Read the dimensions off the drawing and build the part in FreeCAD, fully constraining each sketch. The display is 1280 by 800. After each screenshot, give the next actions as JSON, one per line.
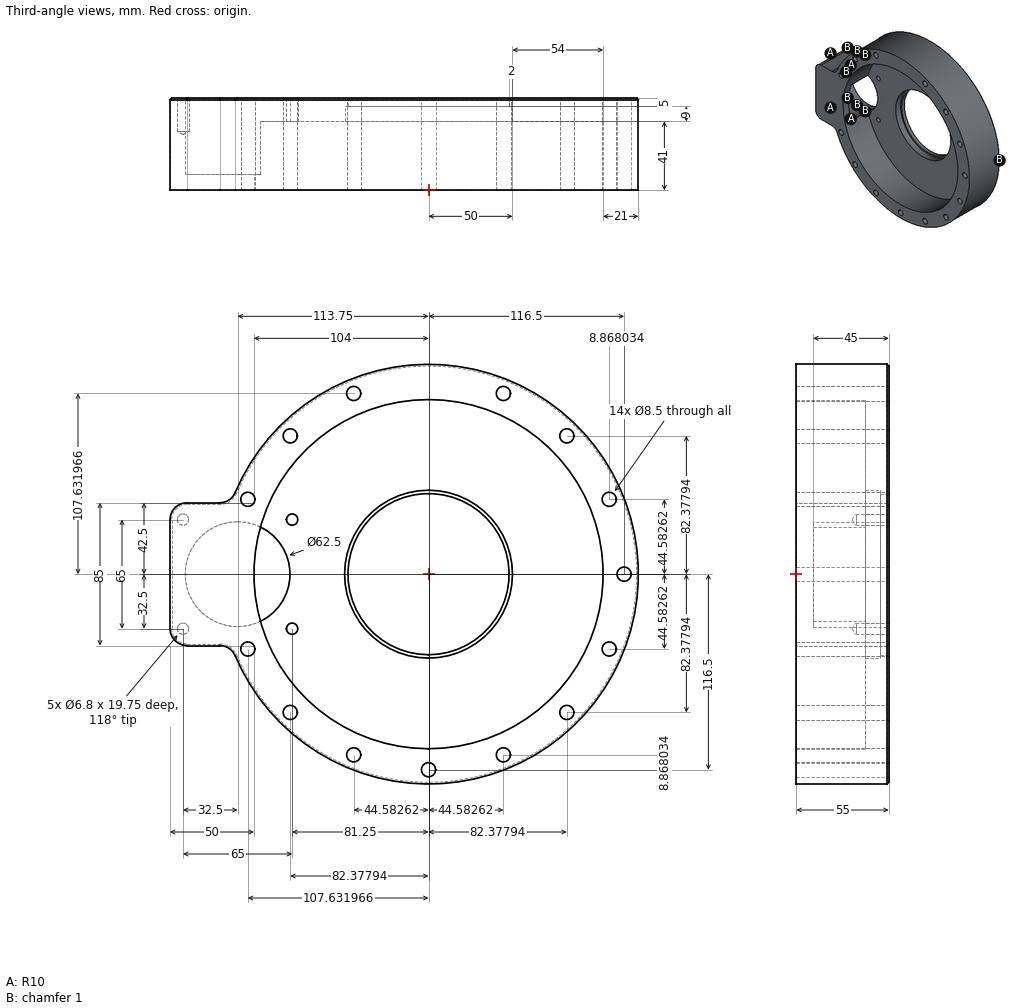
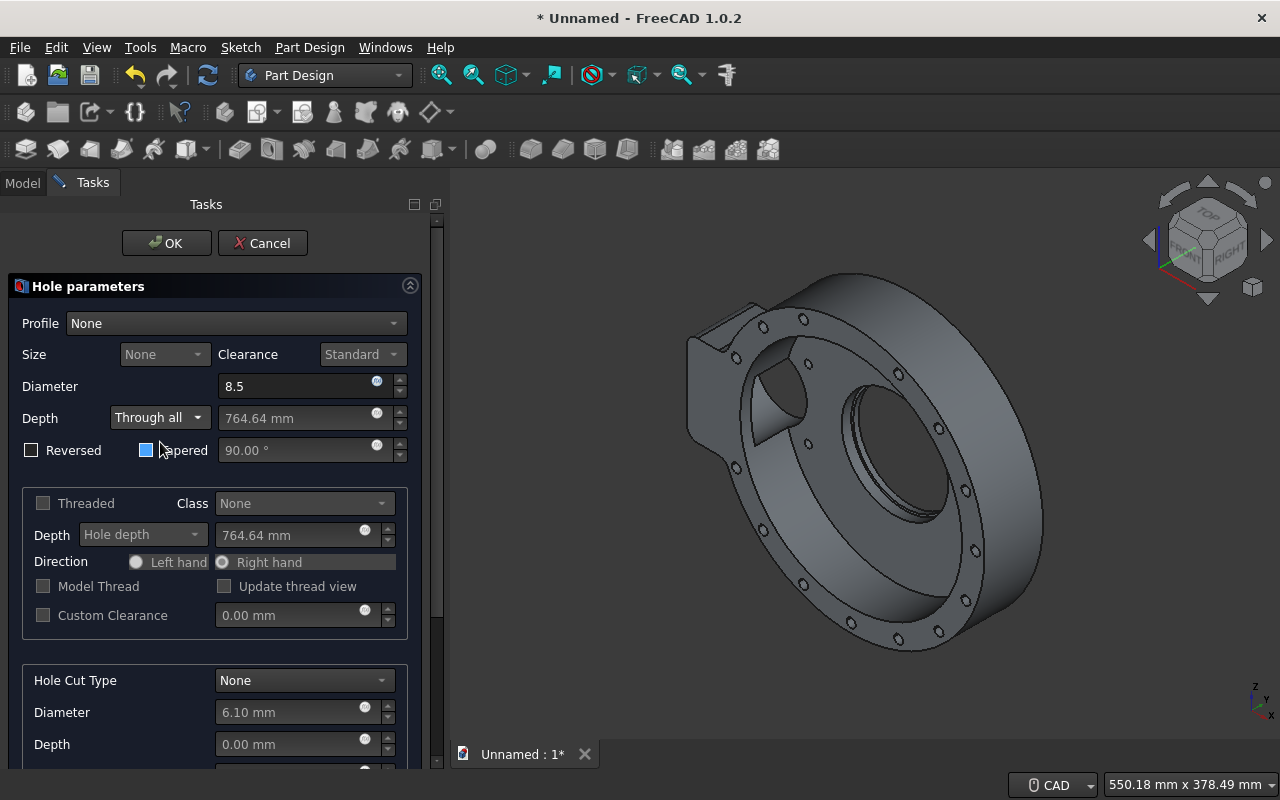
{"action": "left_click", "coordinate": [167, 243]}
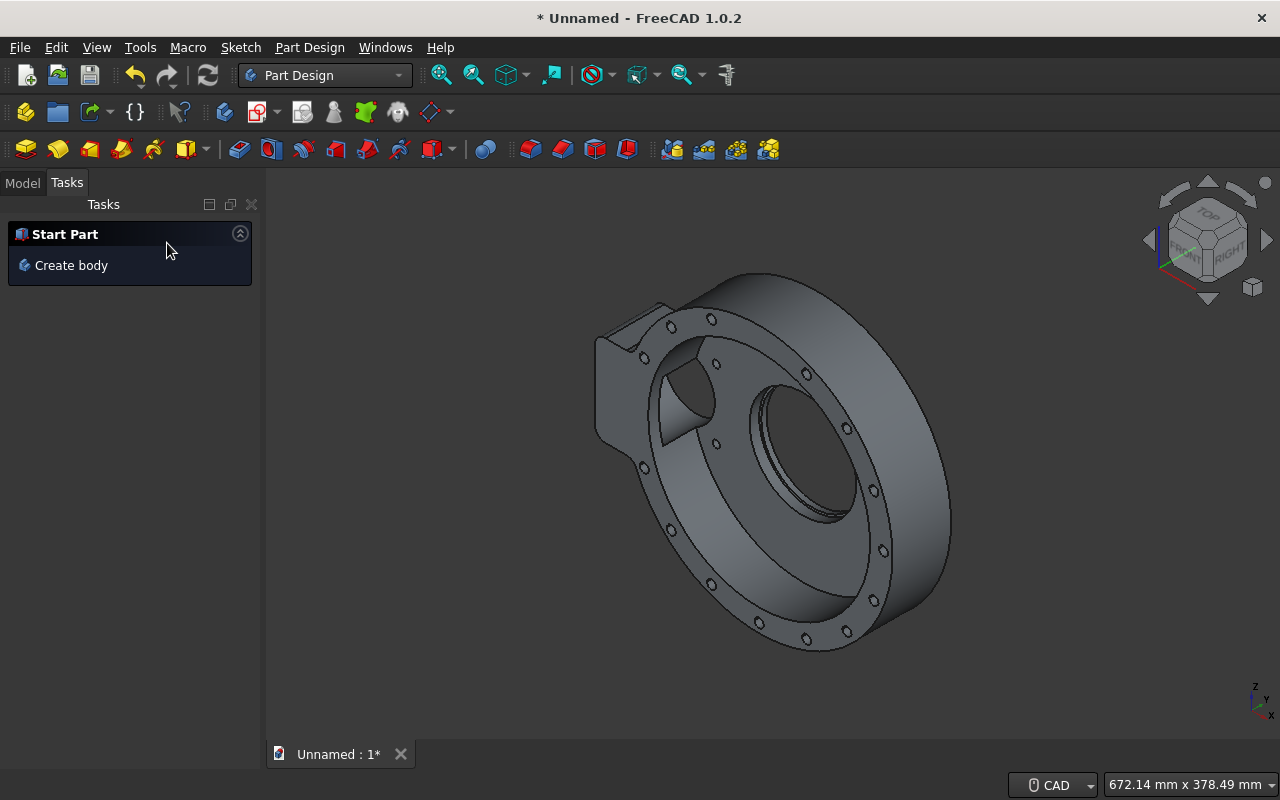
{"action": "key", "text": "2"}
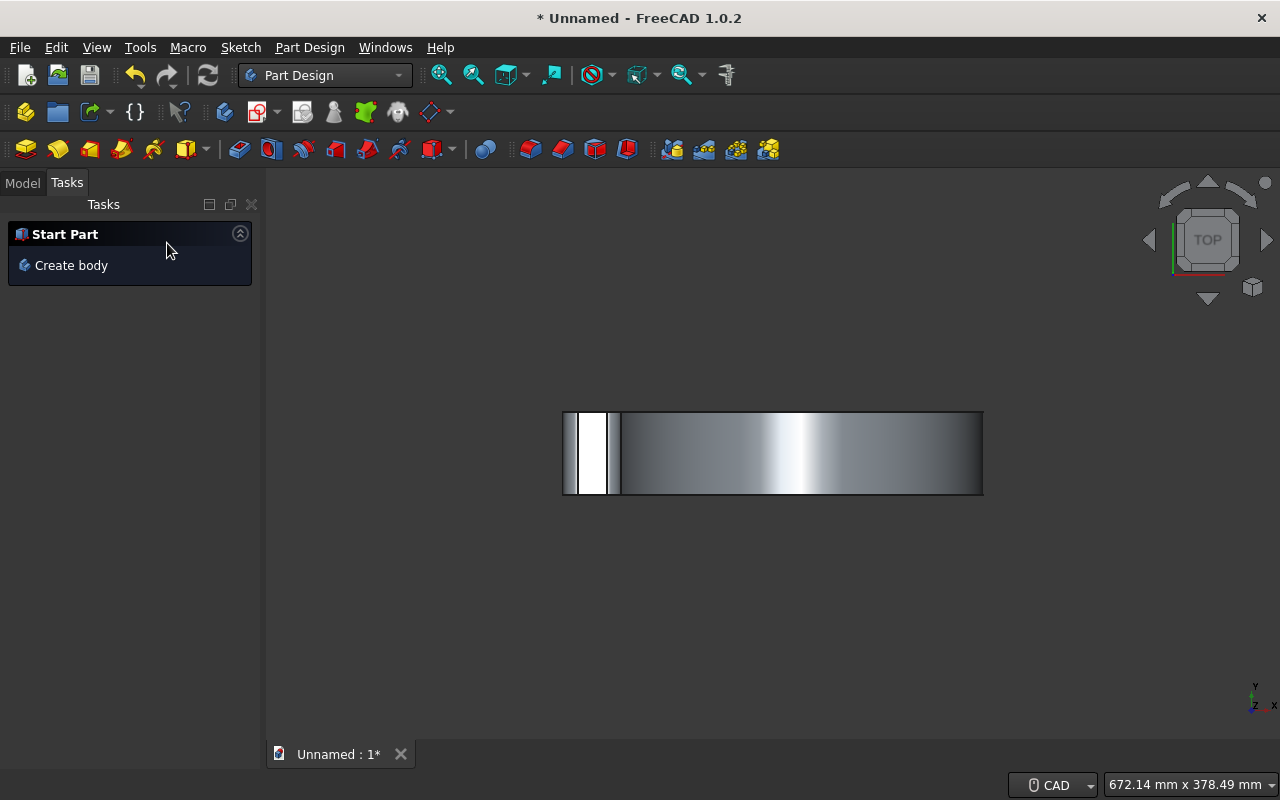
{"action": "left_click", "coordinate": [442, 76]}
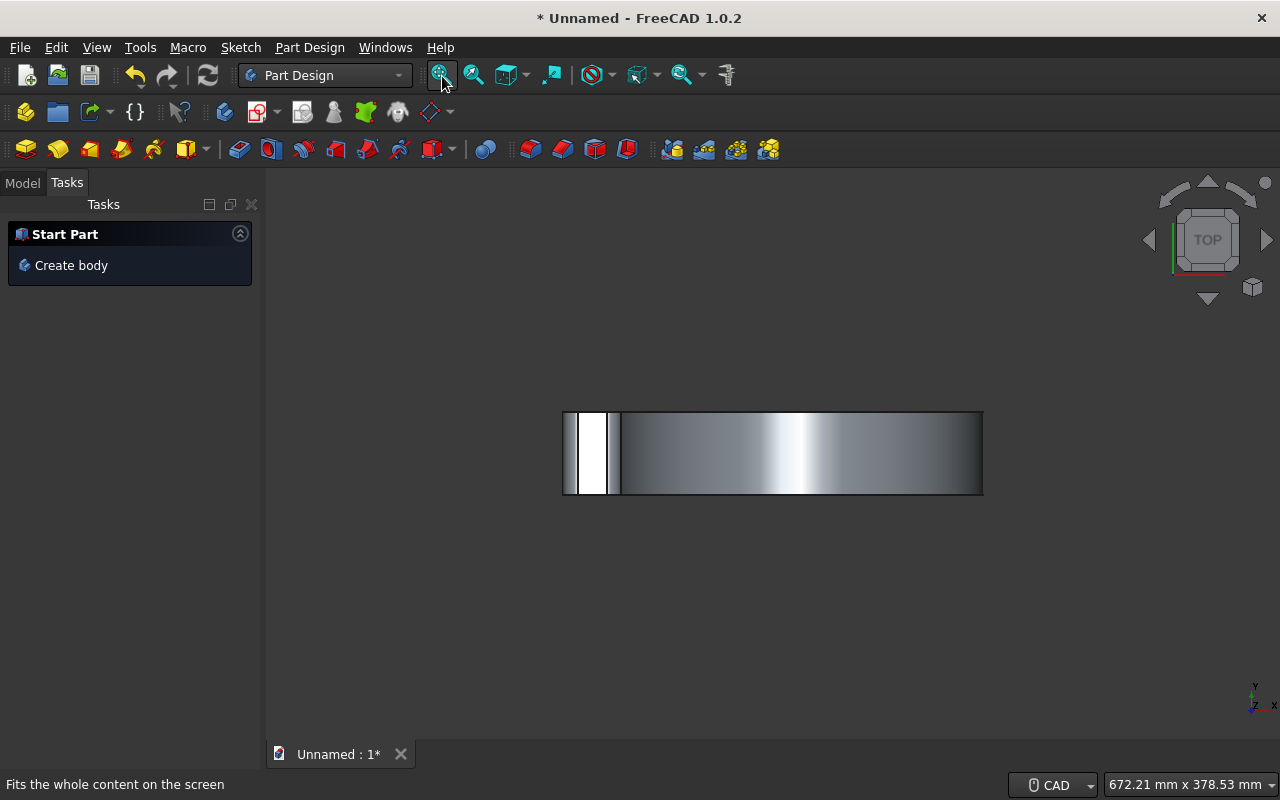
{"action": "left_click", "coordinate": [592, 411]}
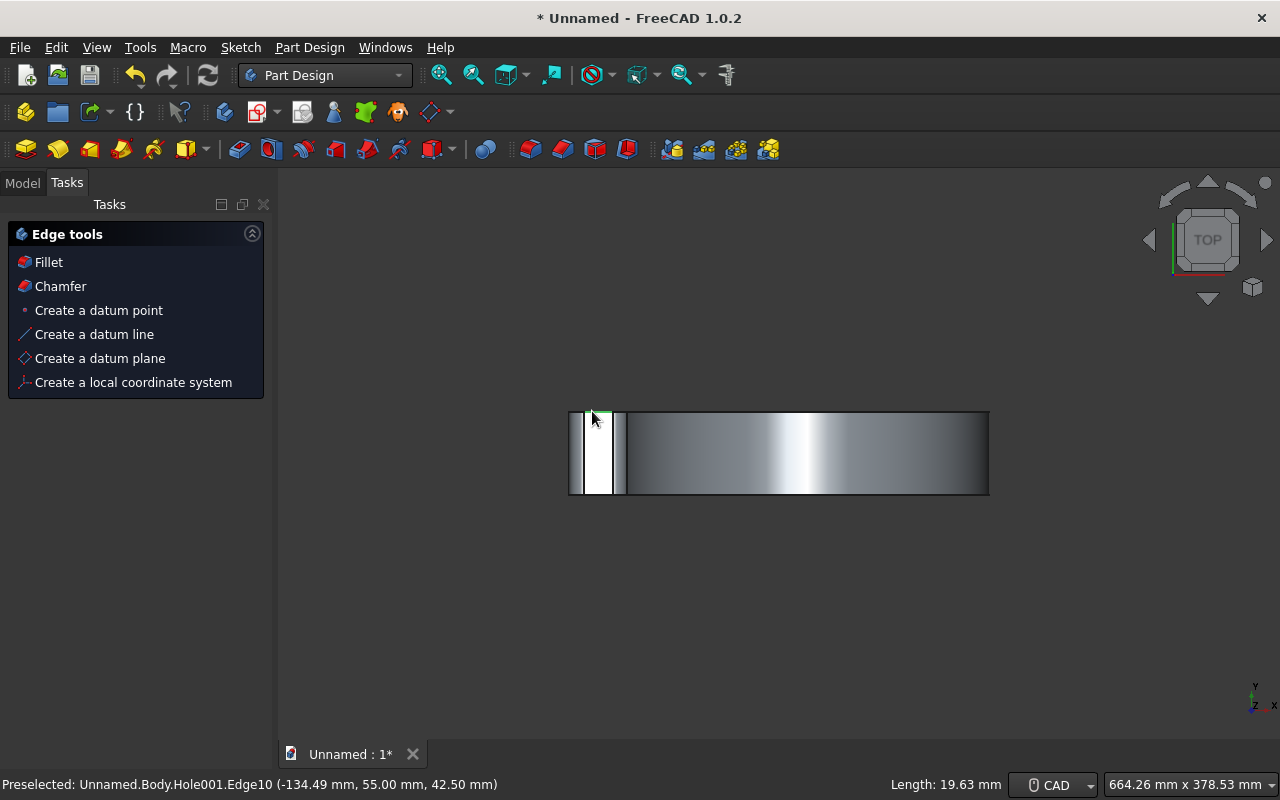
{"action": "left_click", "coordinate": [573, 411], "text": "ctrl"}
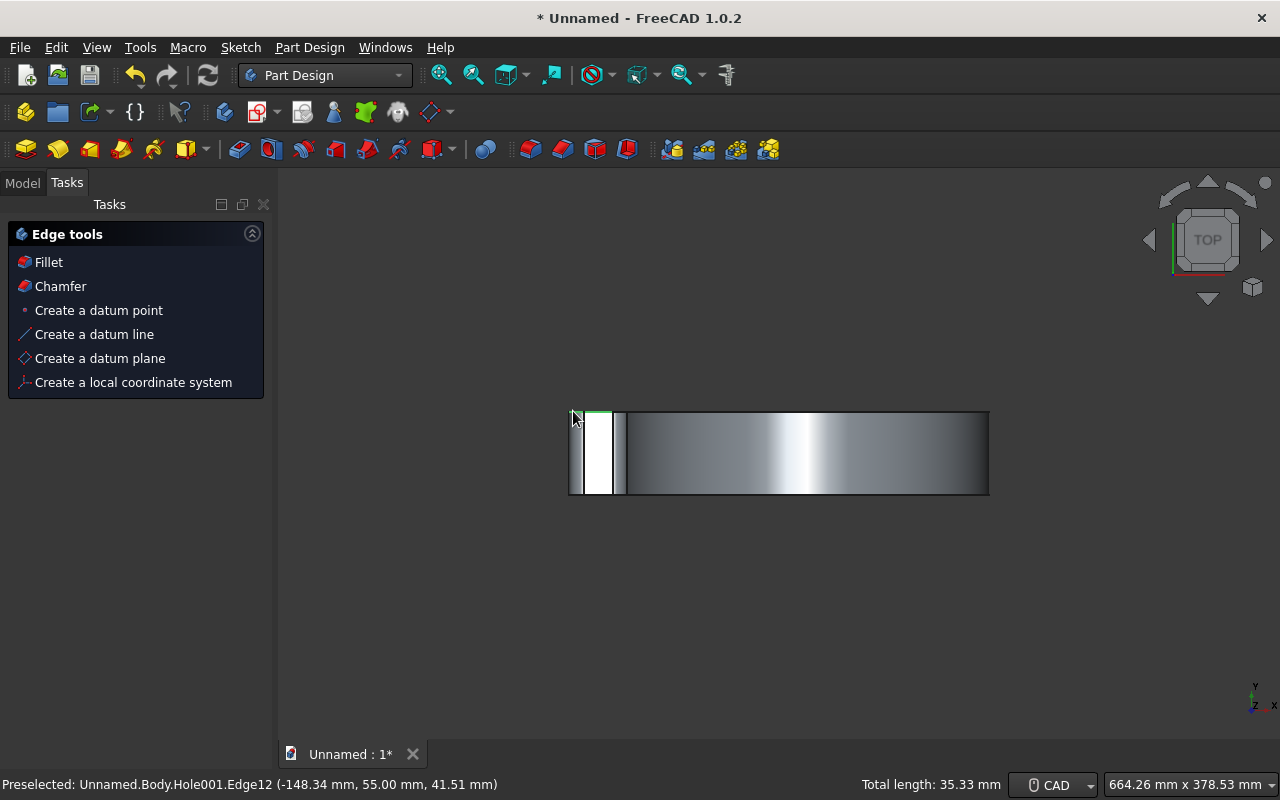
{"action": "left_click", "coordinate": [620, 411], "text": "ctrl"}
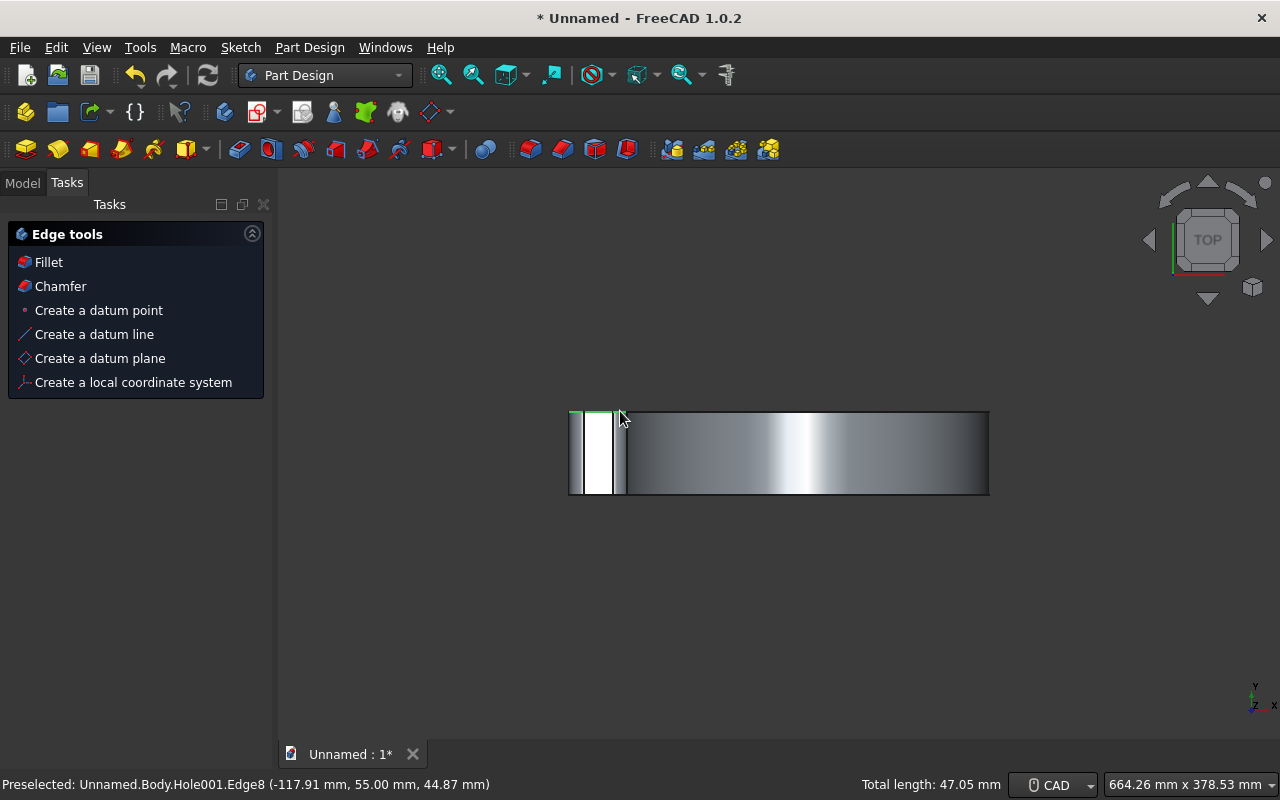
{"action": "key", "text": "0"}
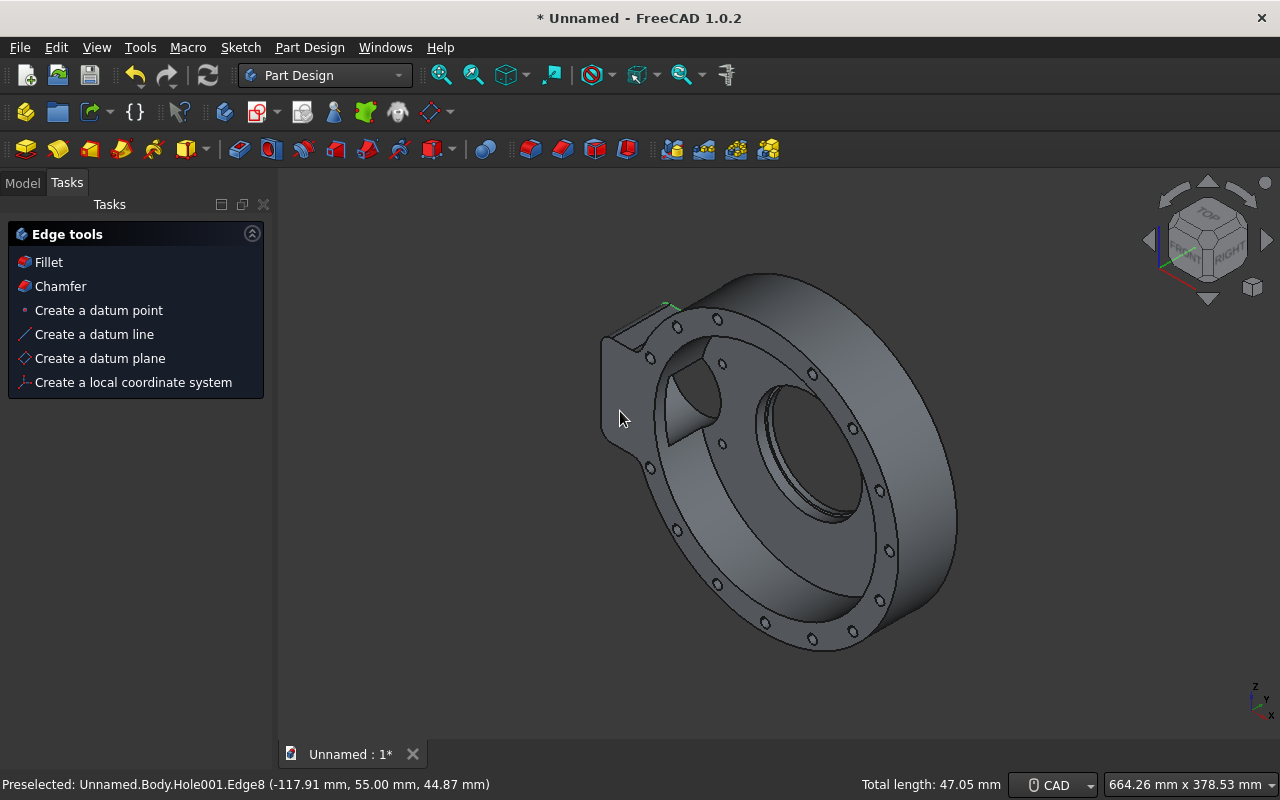
{"action": "key", "text": "1"}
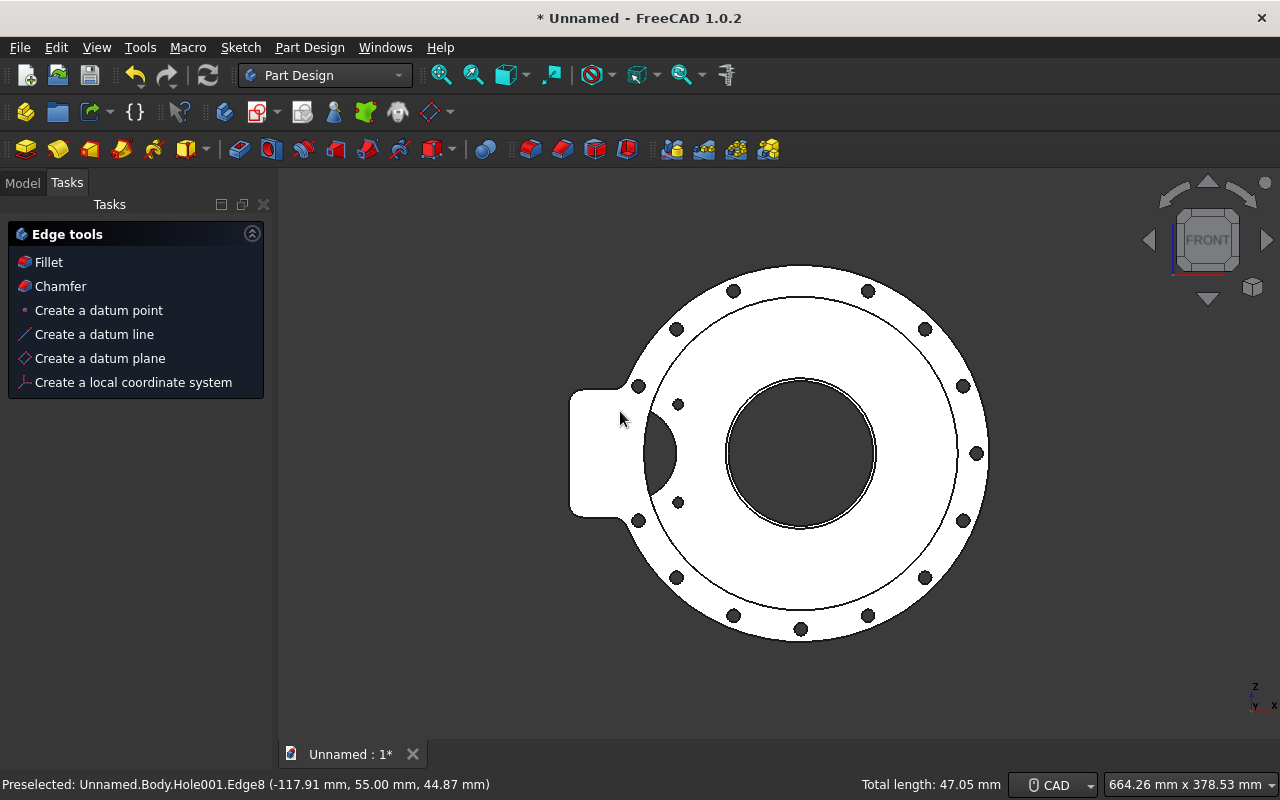
{"action": "key", "text": "3"}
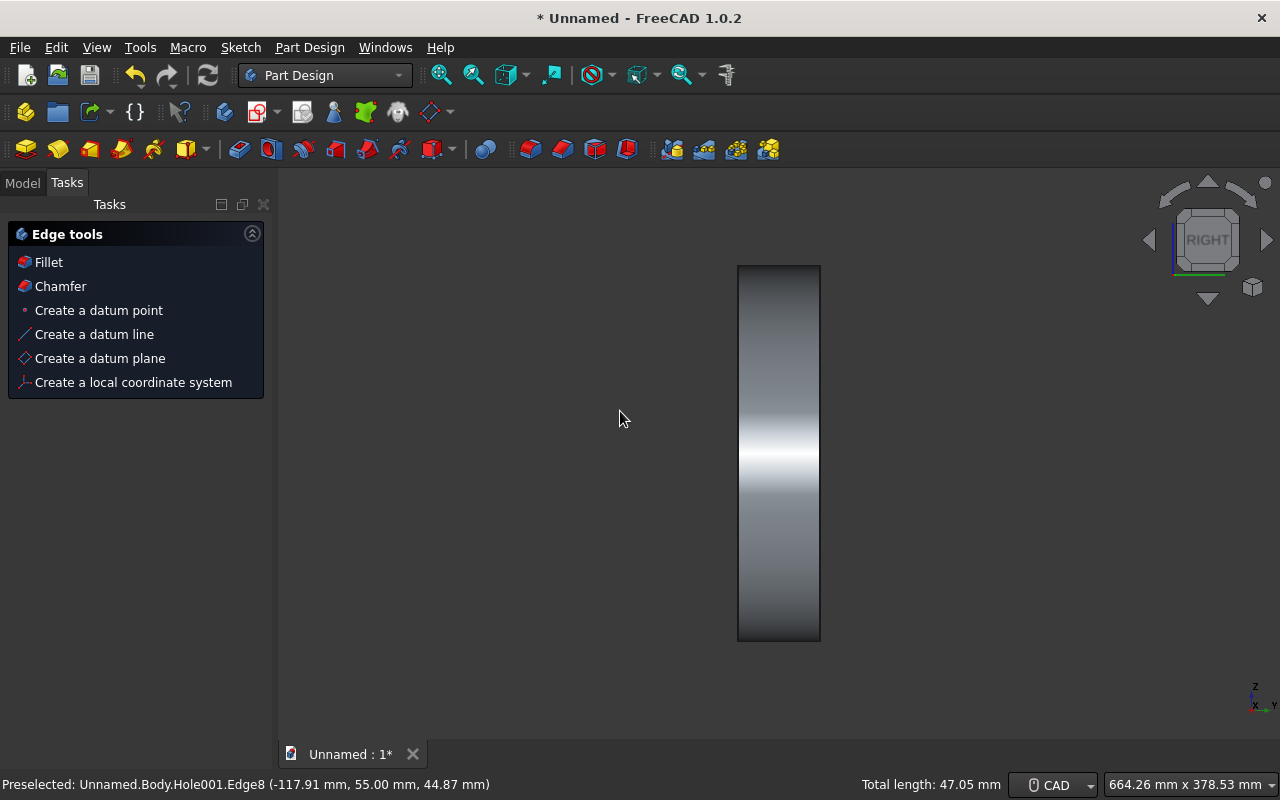
{"action": "left_click", "coordinate": [820, 637], "text": "ctrl"}